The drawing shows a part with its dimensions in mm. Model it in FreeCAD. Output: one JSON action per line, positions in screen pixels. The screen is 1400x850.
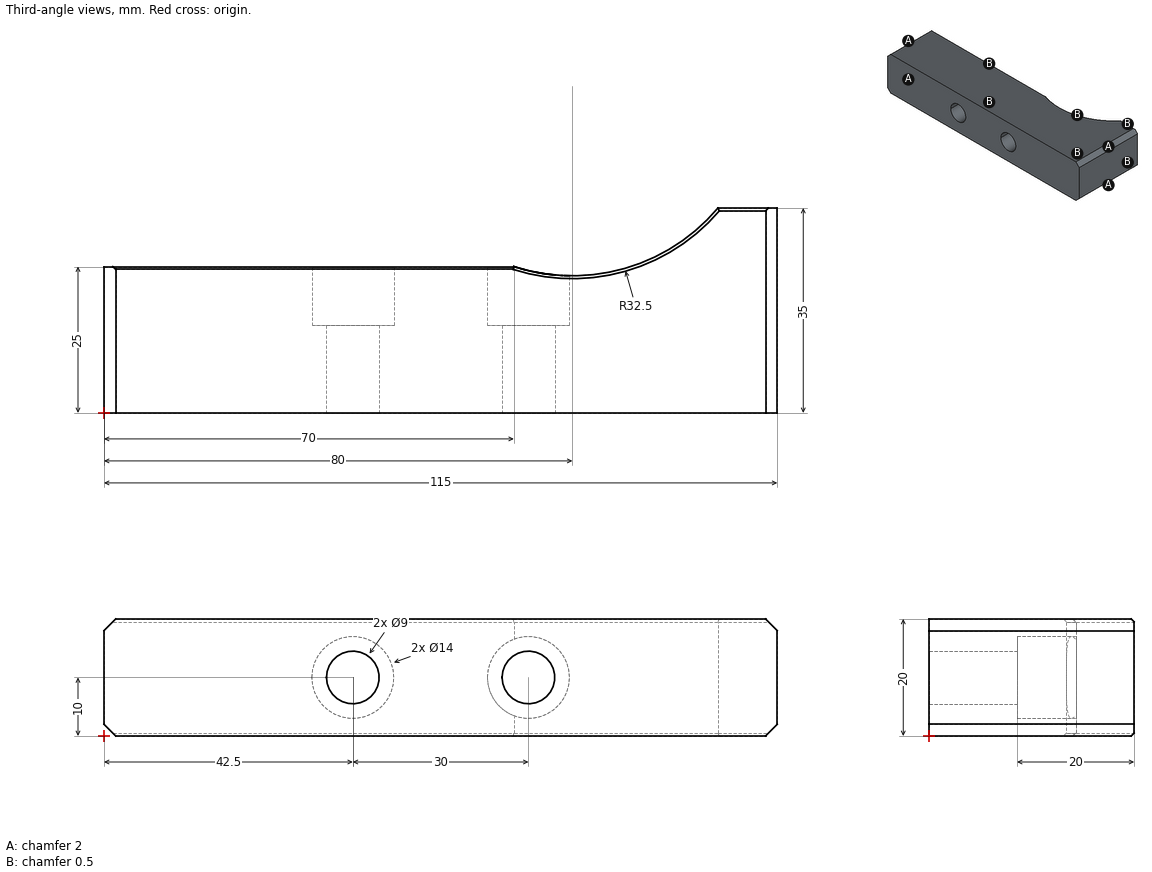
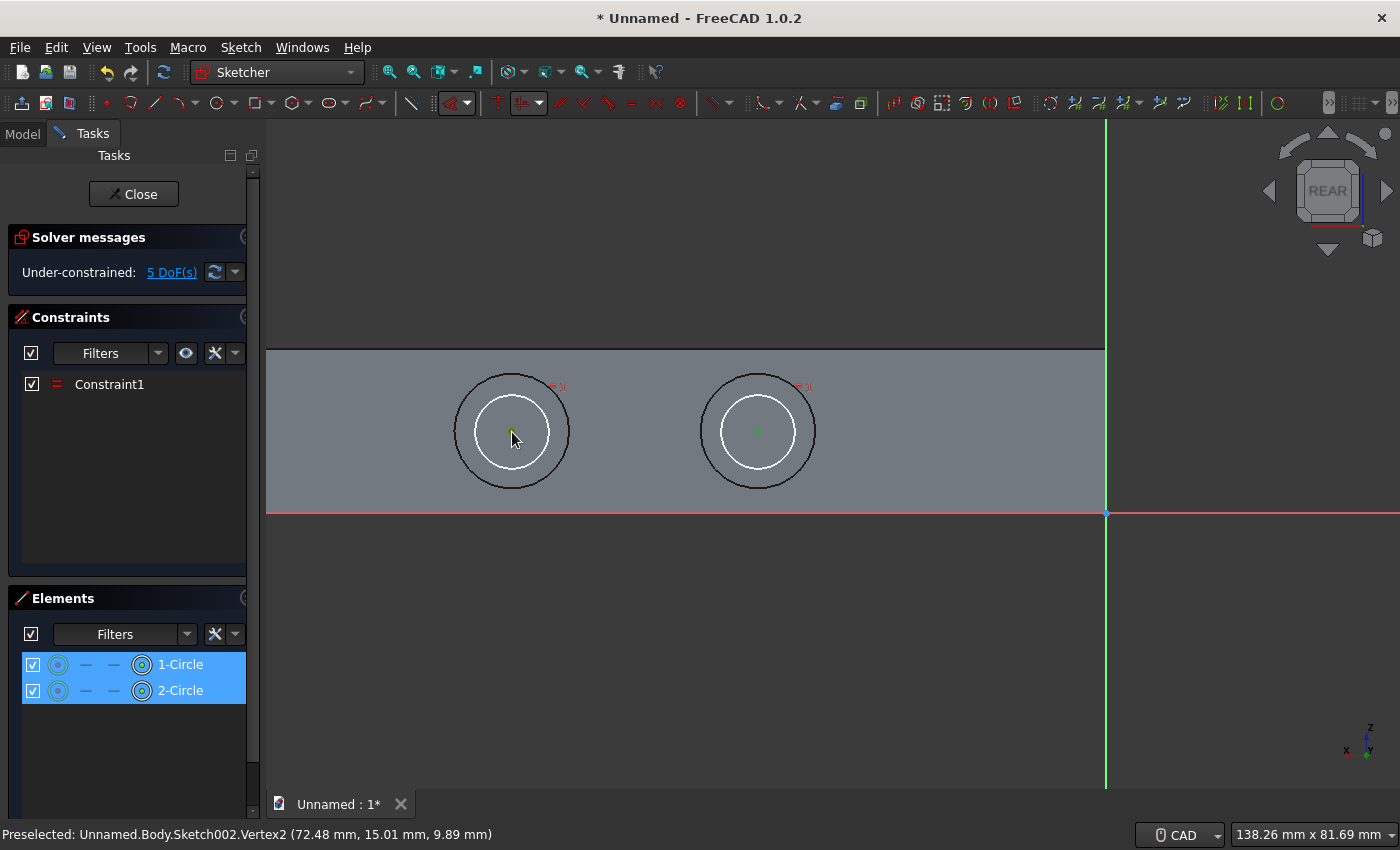
{"action": "key", "text": "h"}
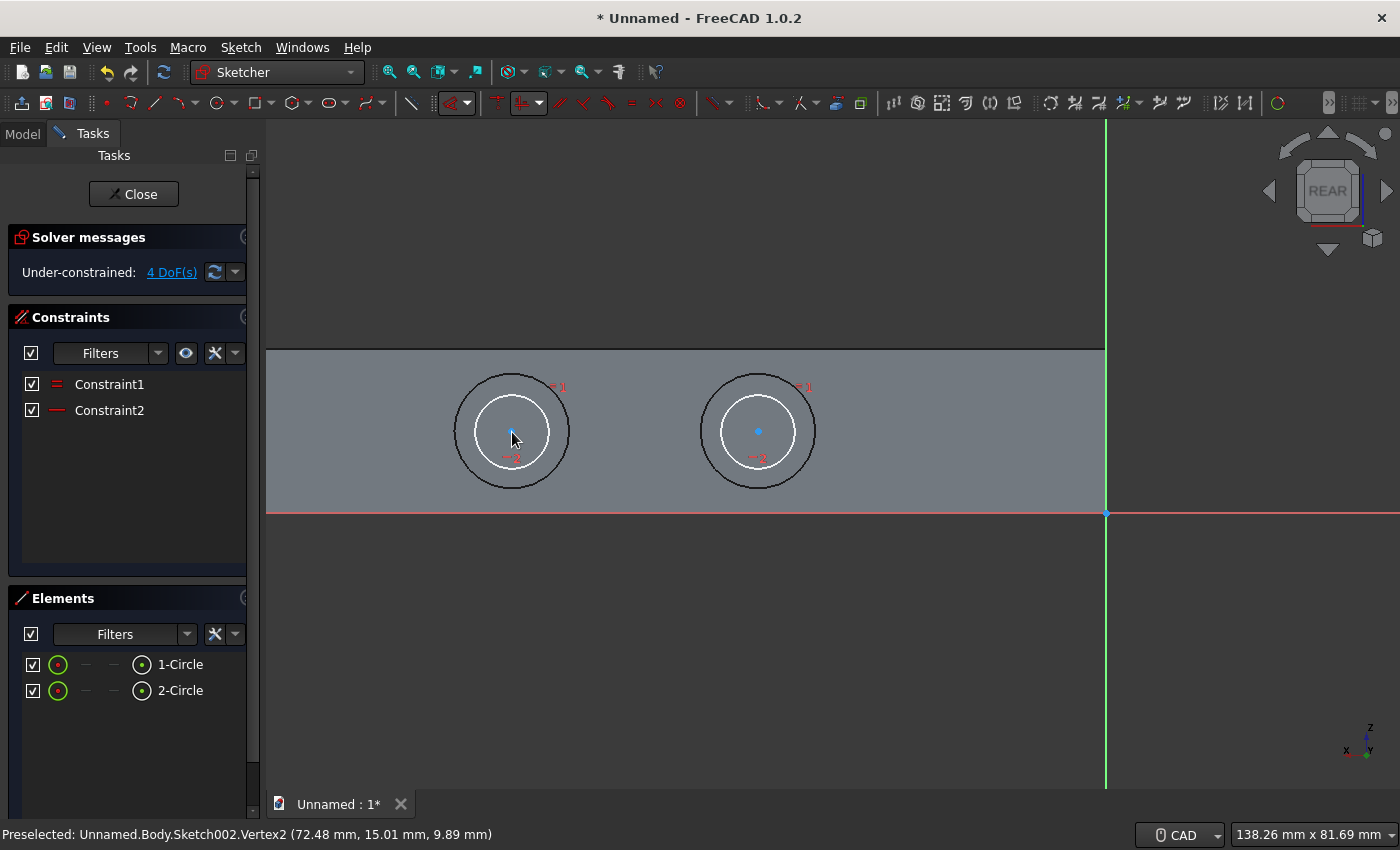
{"action": "left_click", "coordinate": [784, 406]}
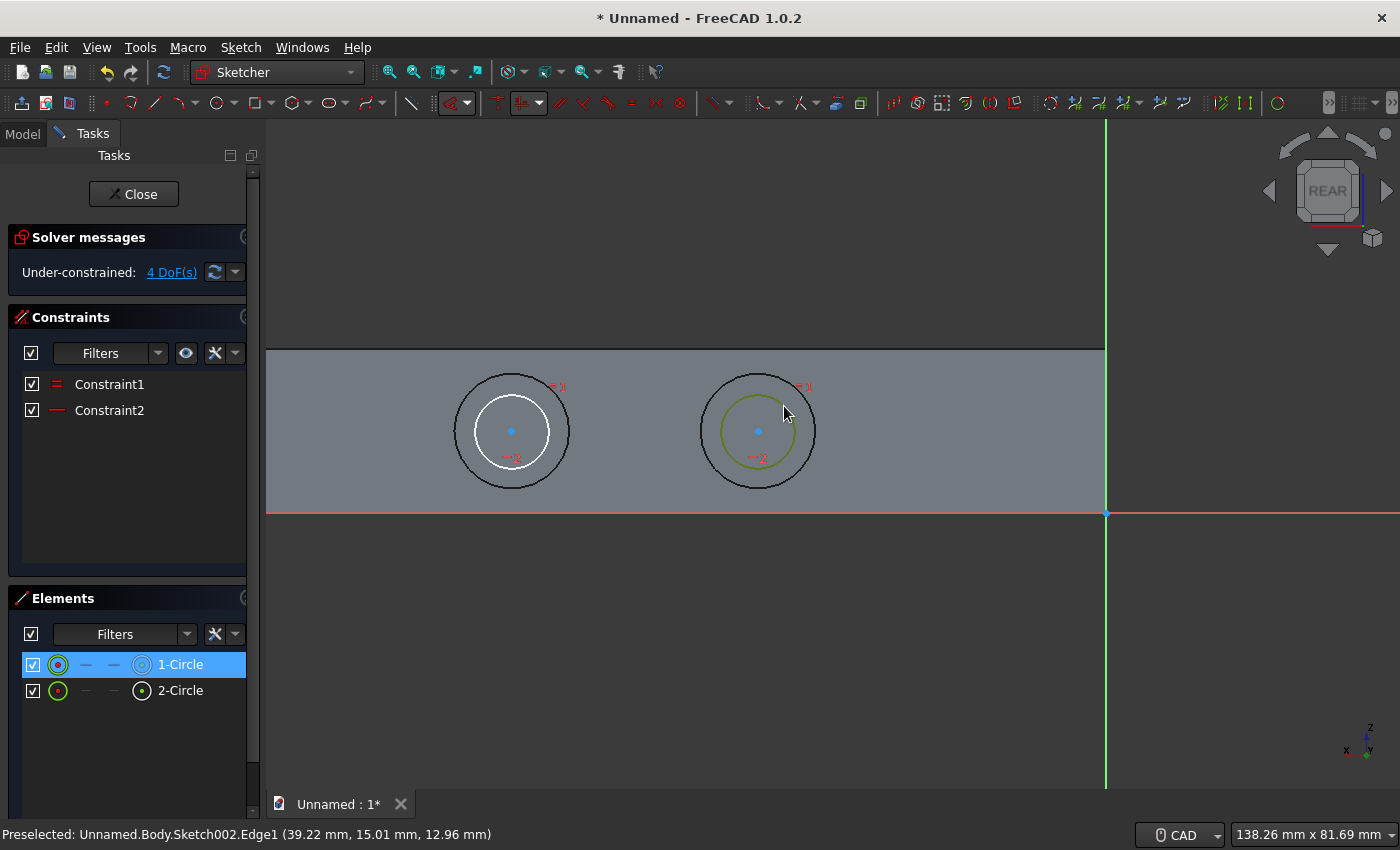
{"action": "left_click", "coordinate": [470, 104]}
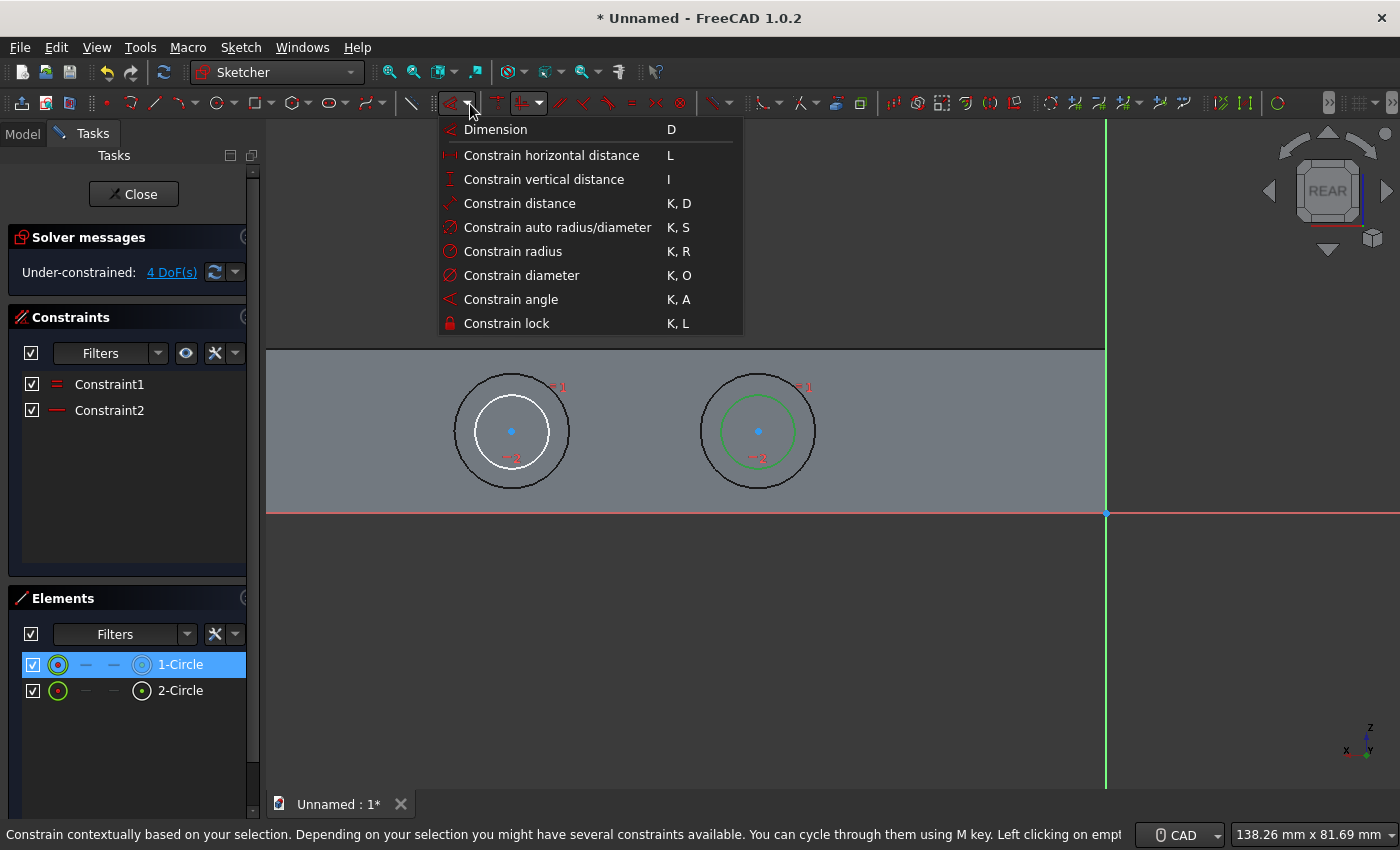
{"action": "left_click", "coordinate": [591, 275]}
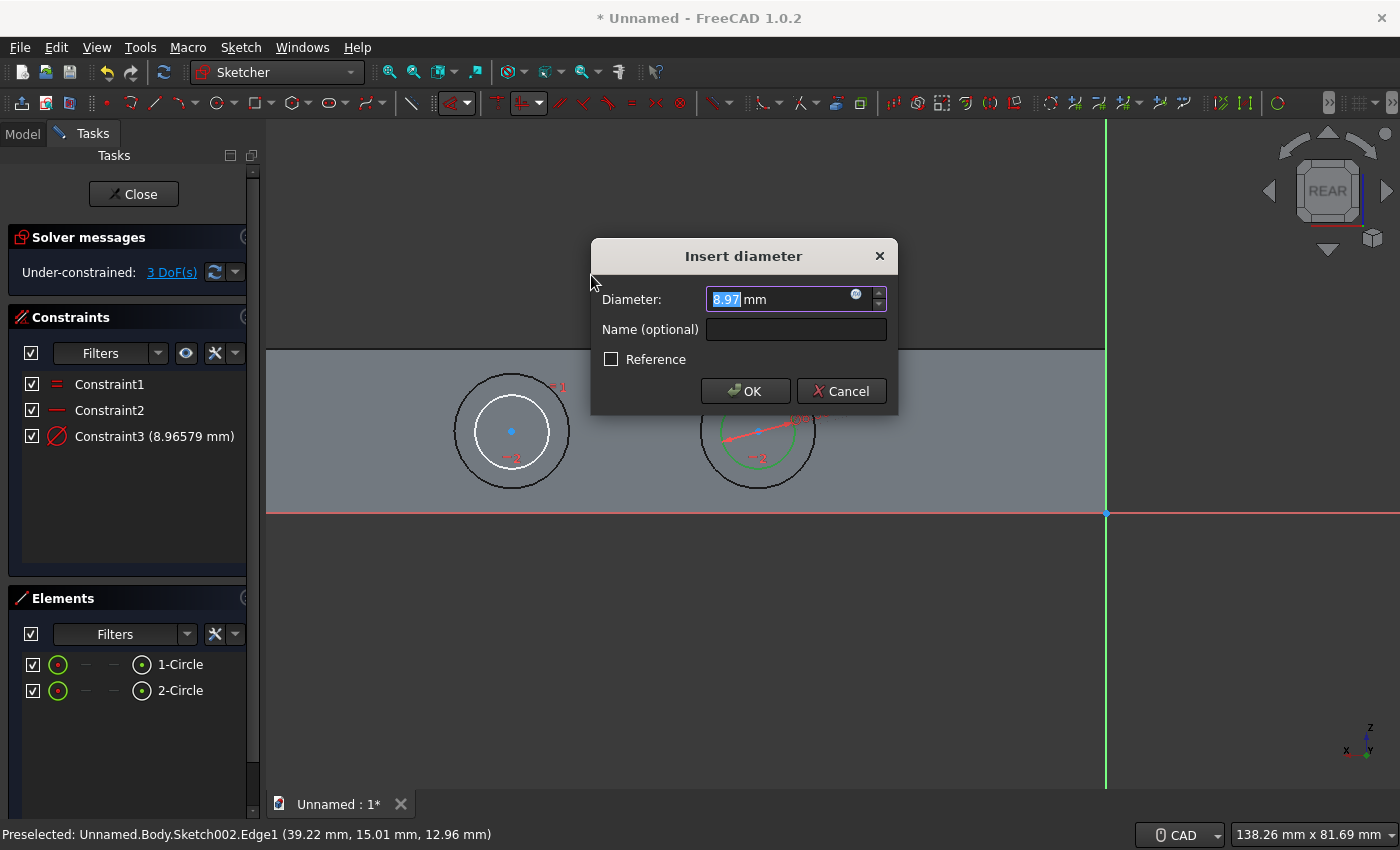
{"action": "type", "text": "9"}
{"action": "key", "text": "Return"}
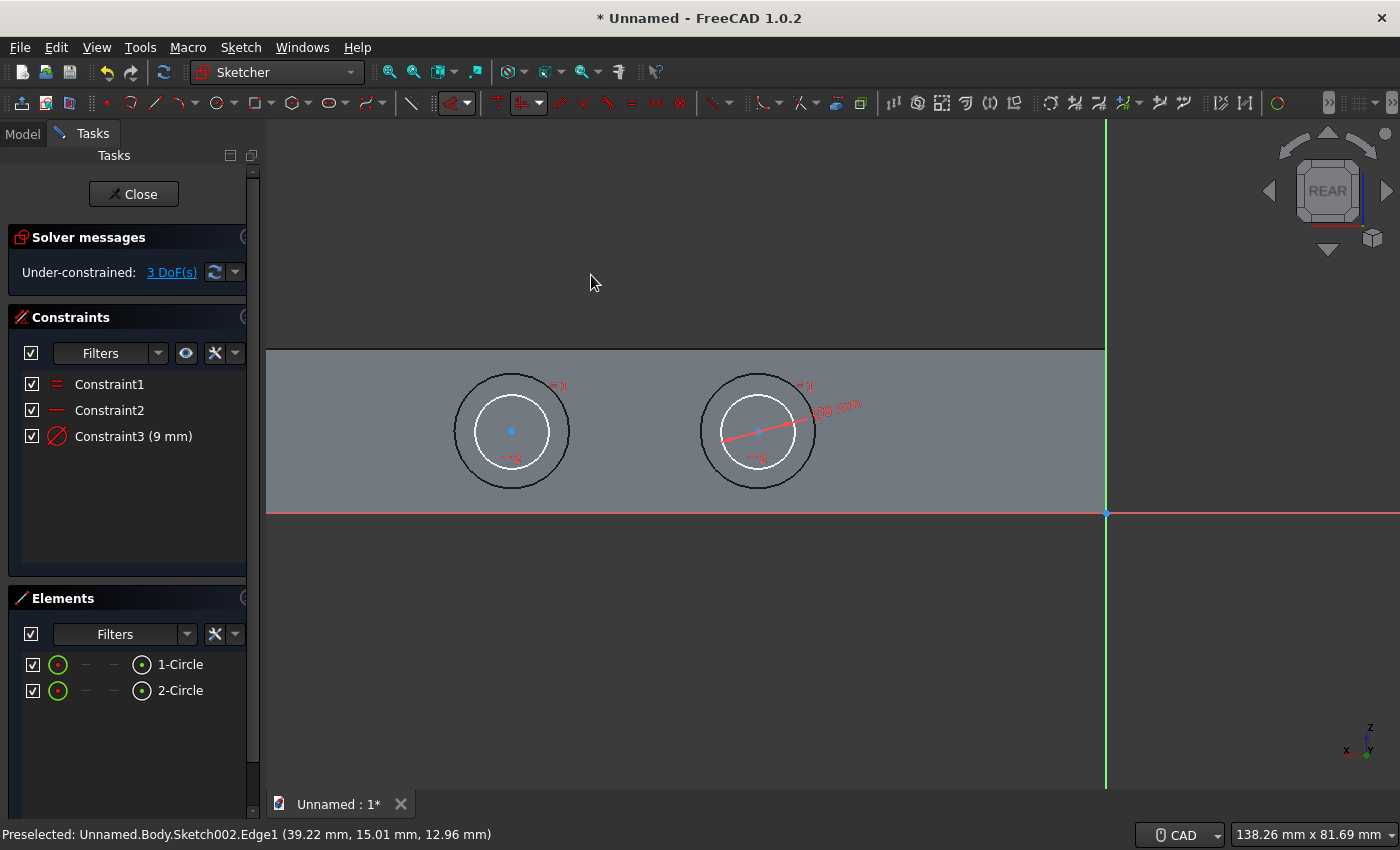
{"action": "left_click", "coordinate": [758, 432]}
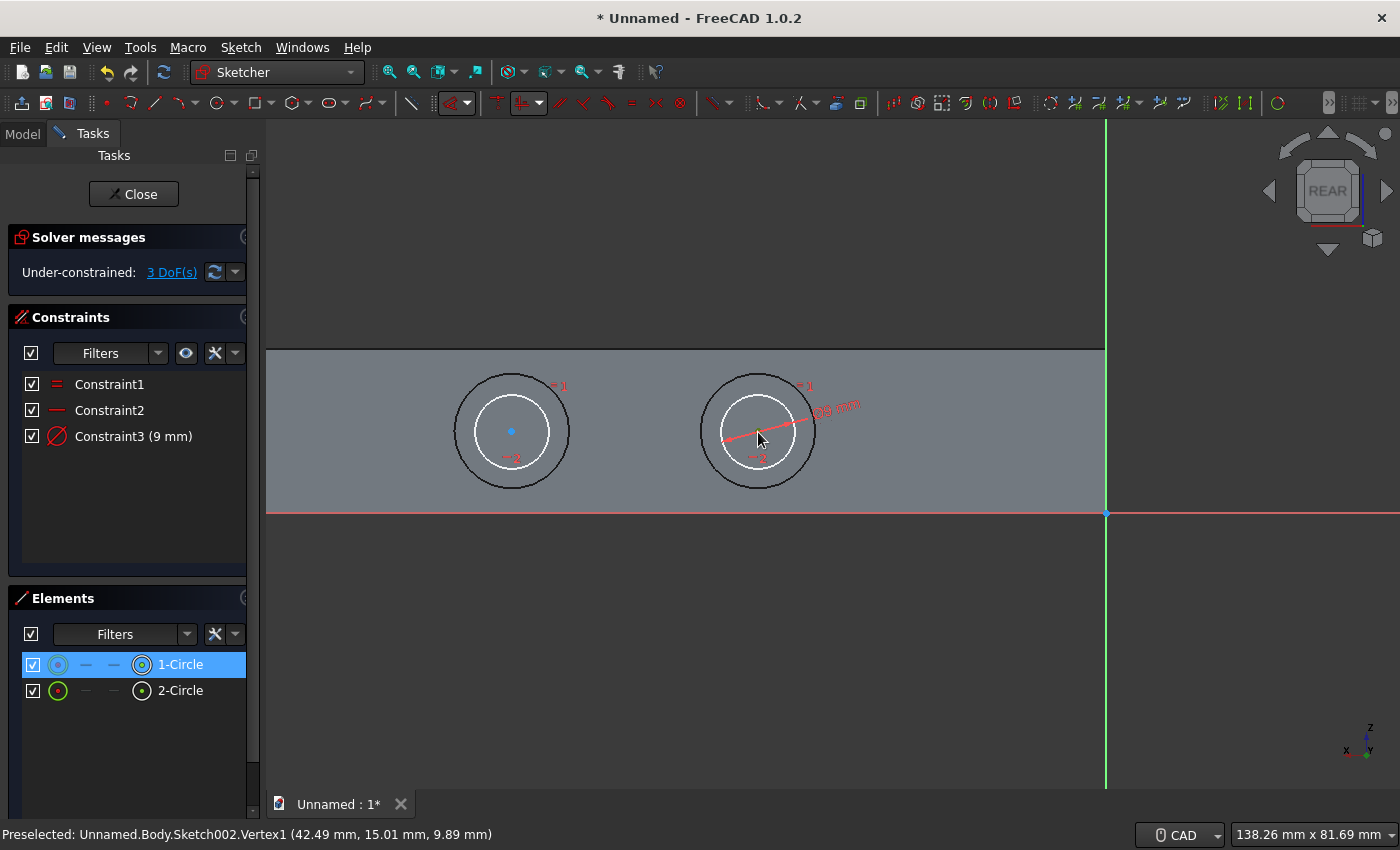
{"action": "key", "text": "i"}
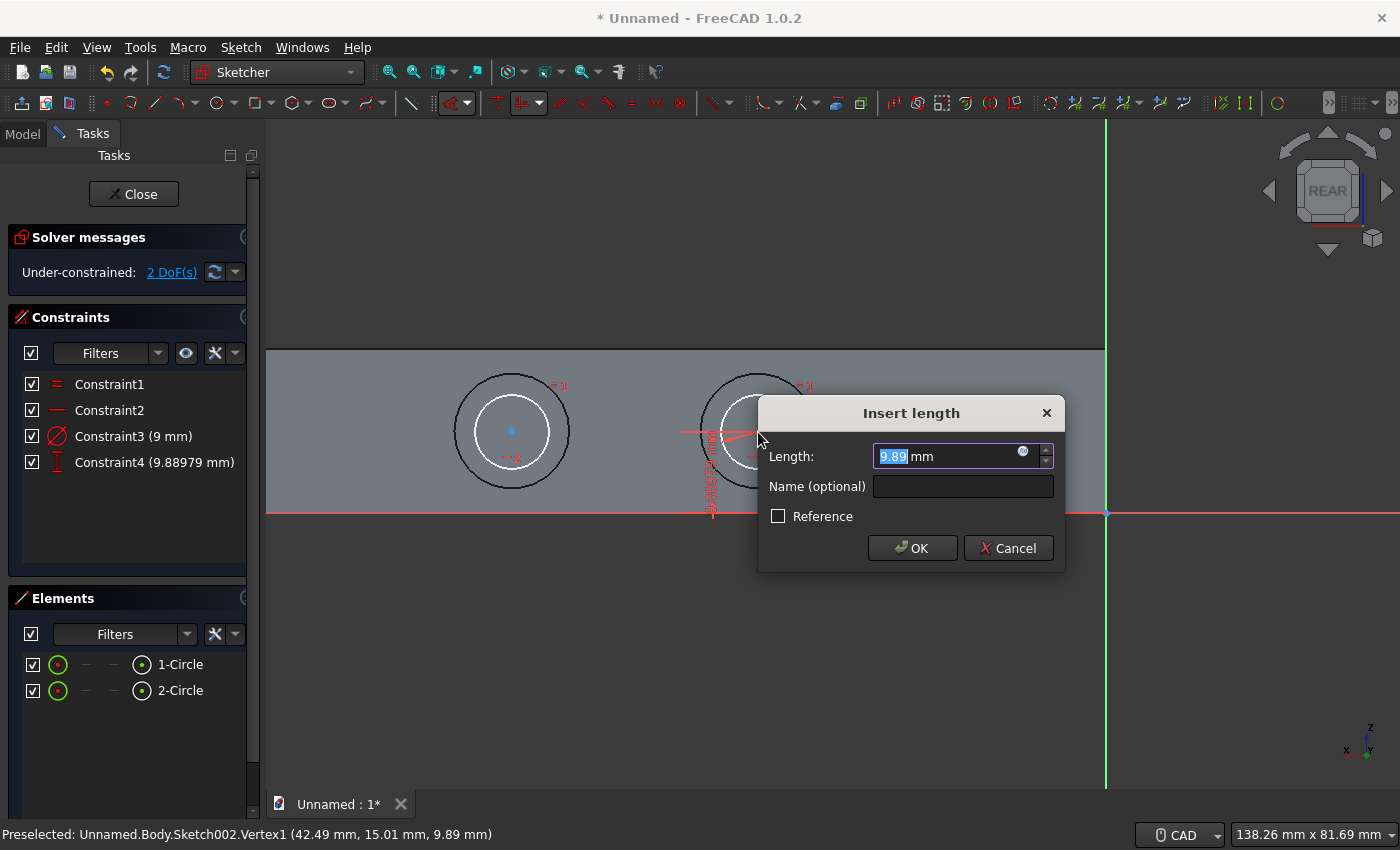
{"action": "type", "text": "10"}
{"action": "key", "text": "Return"}